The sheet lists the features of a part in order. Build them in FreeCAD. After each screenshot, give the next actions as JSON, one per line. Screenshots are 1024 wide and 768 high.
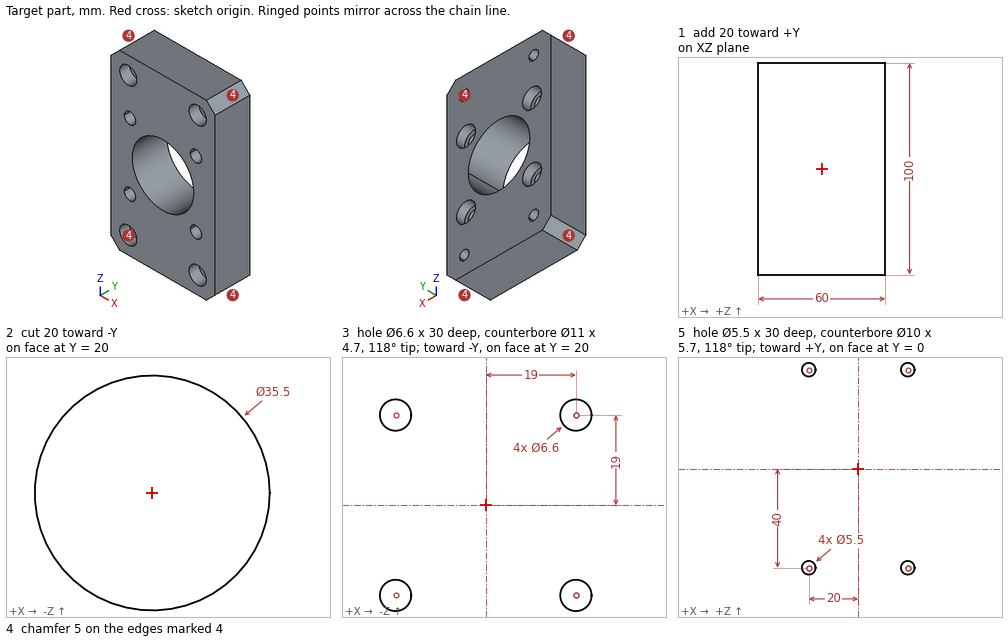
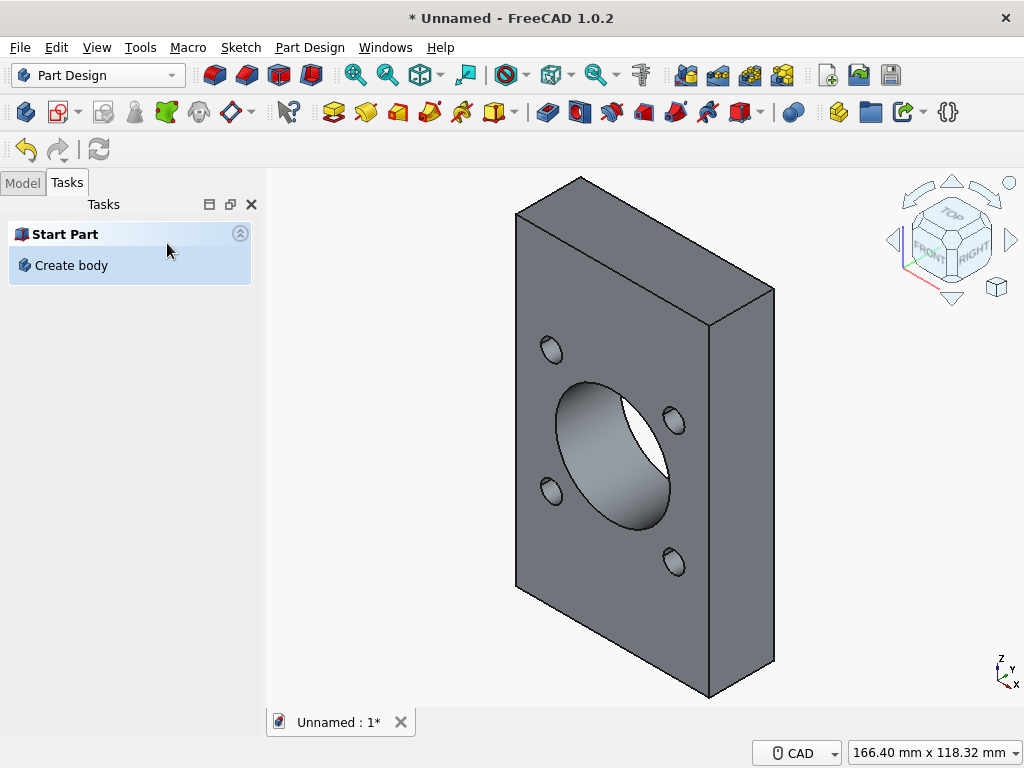
{"action": "left_click", "coordinate": [742, 306]}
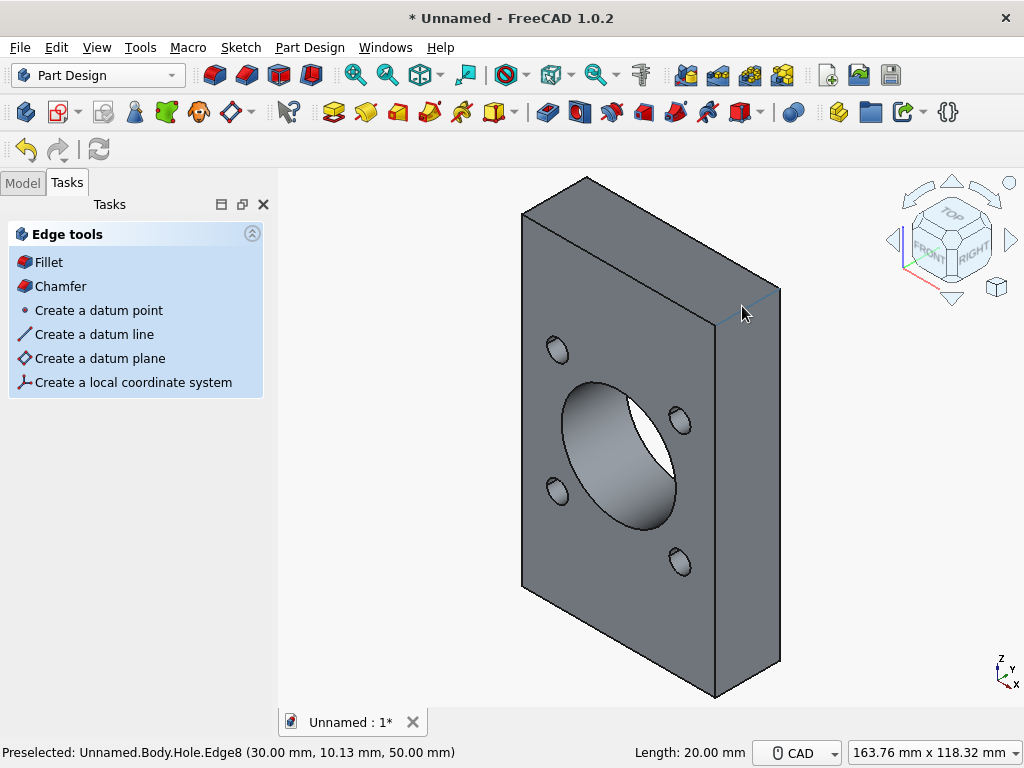
{"action": "key", "text": "2"}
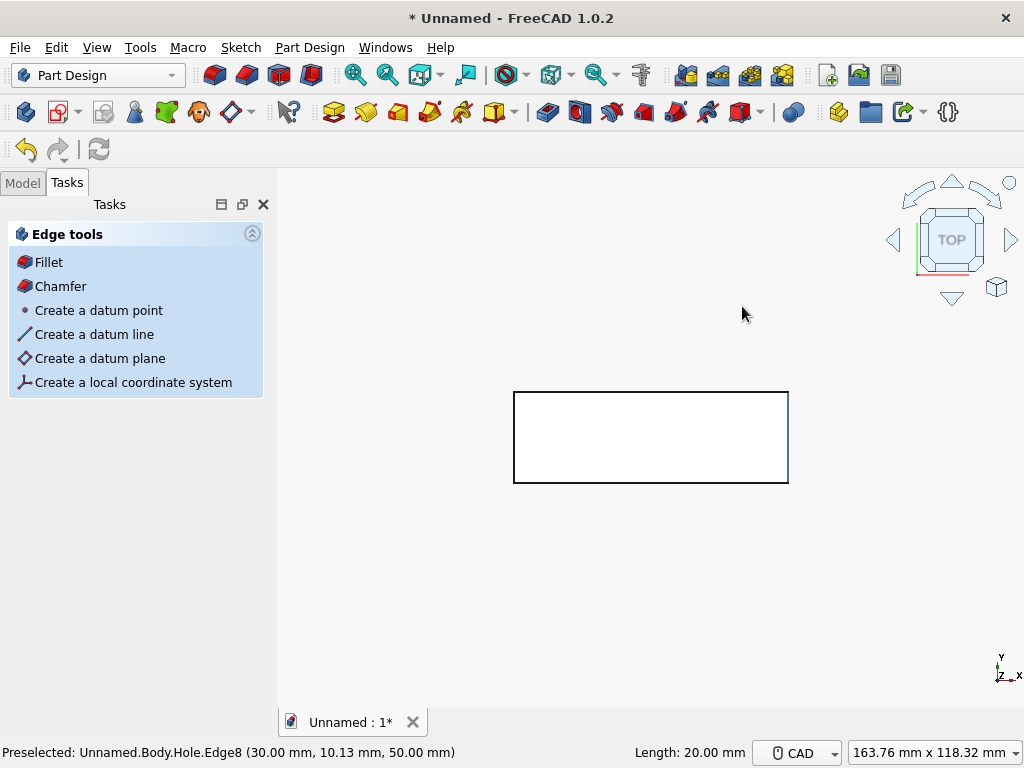
{"action": "left_click", "coordinate": [356, 76]}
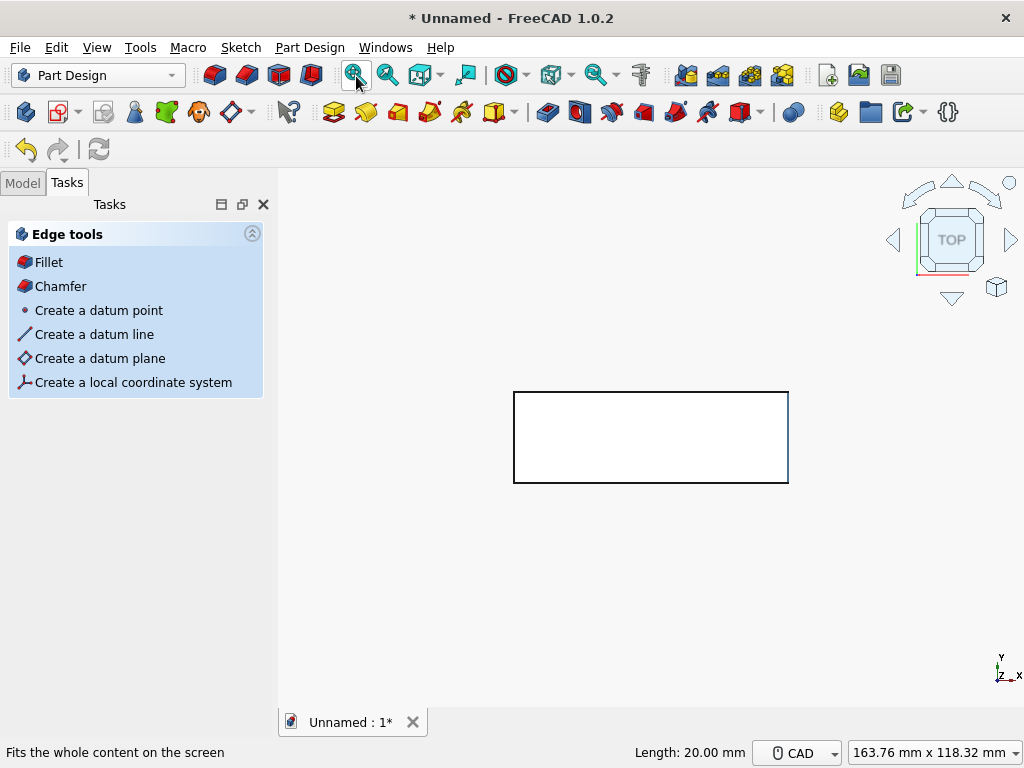
{"action": "left_click", "coordinate": [514, 436], "text": "ctrl"}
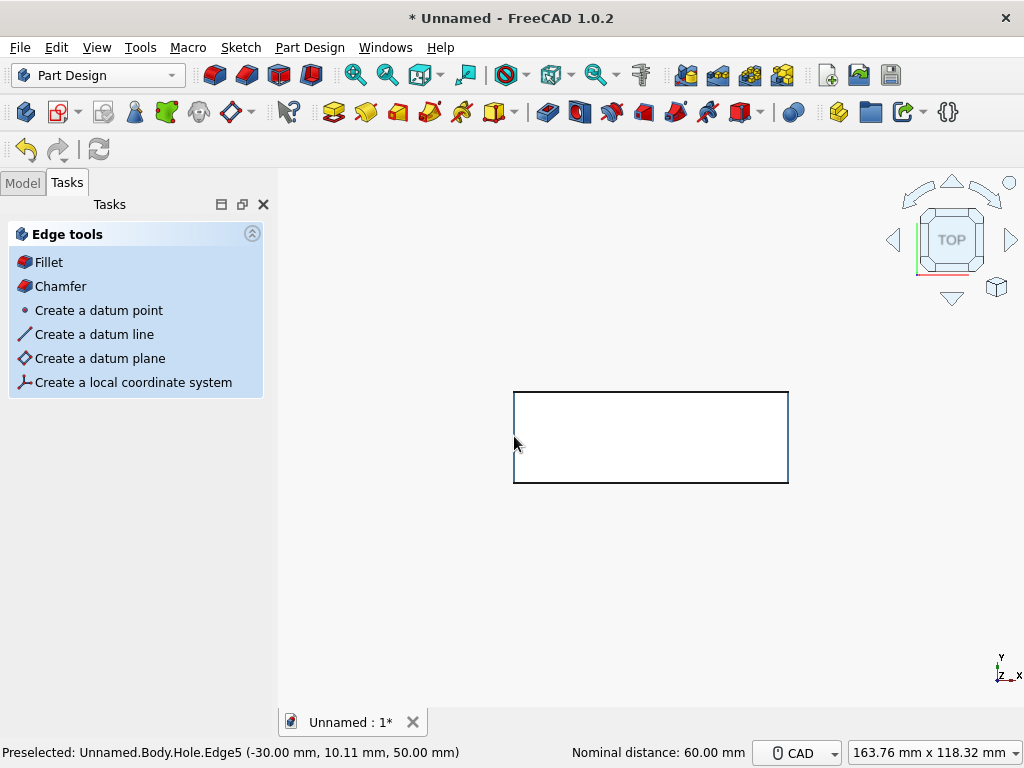
{"action": "key", "text": "1"}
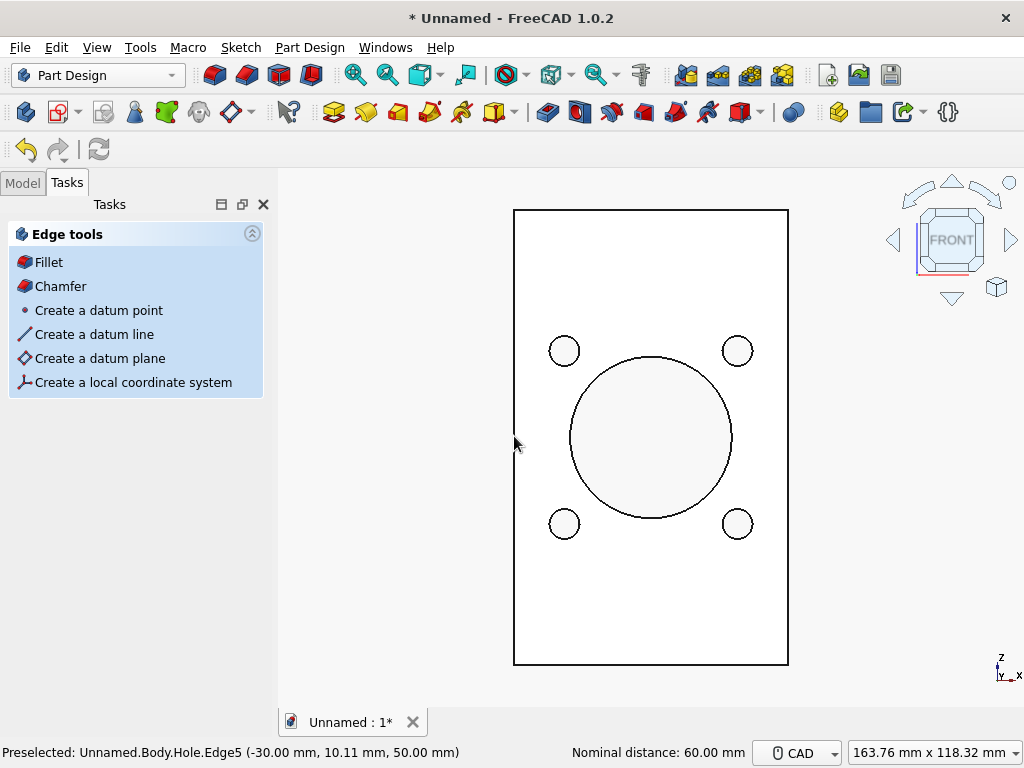
{"action": "key", "text": "3"}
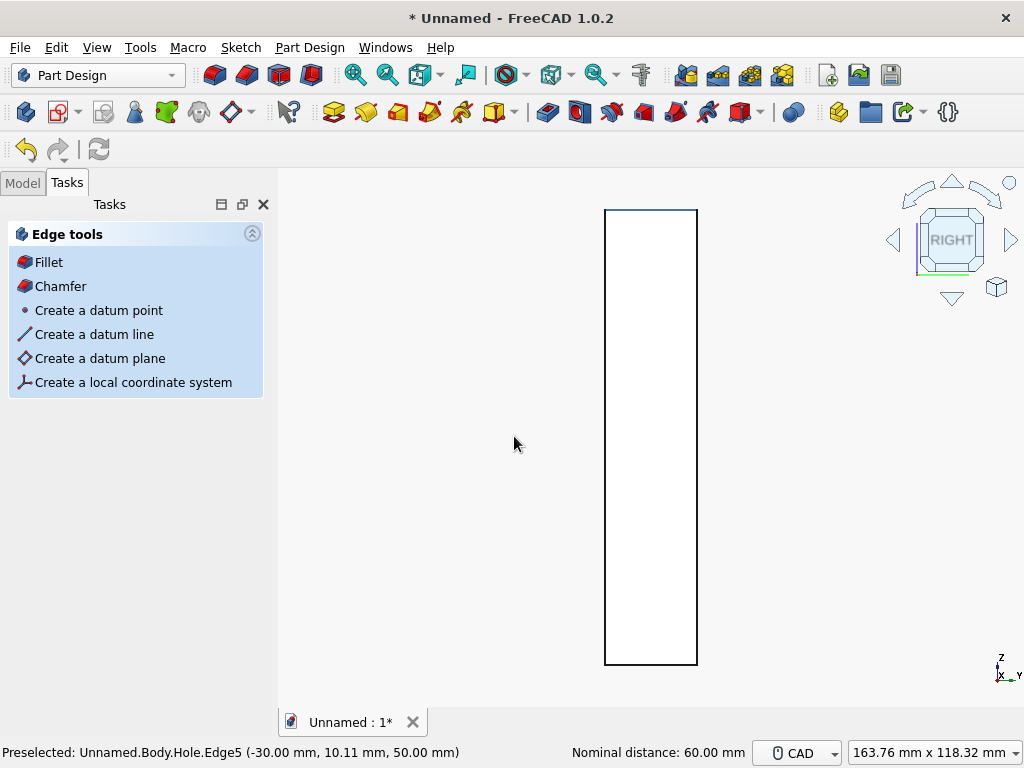
{"action": "left_click", "coordinate": [651, 664], "text": "ctrl"}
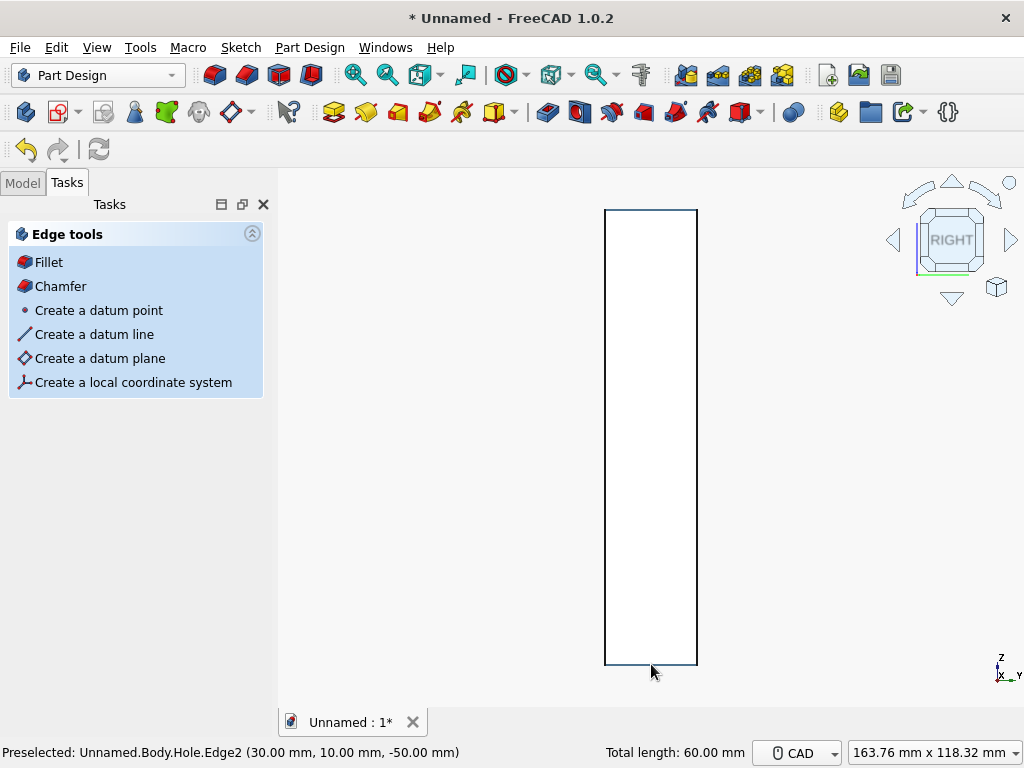
{"action": "key", "text": "5"}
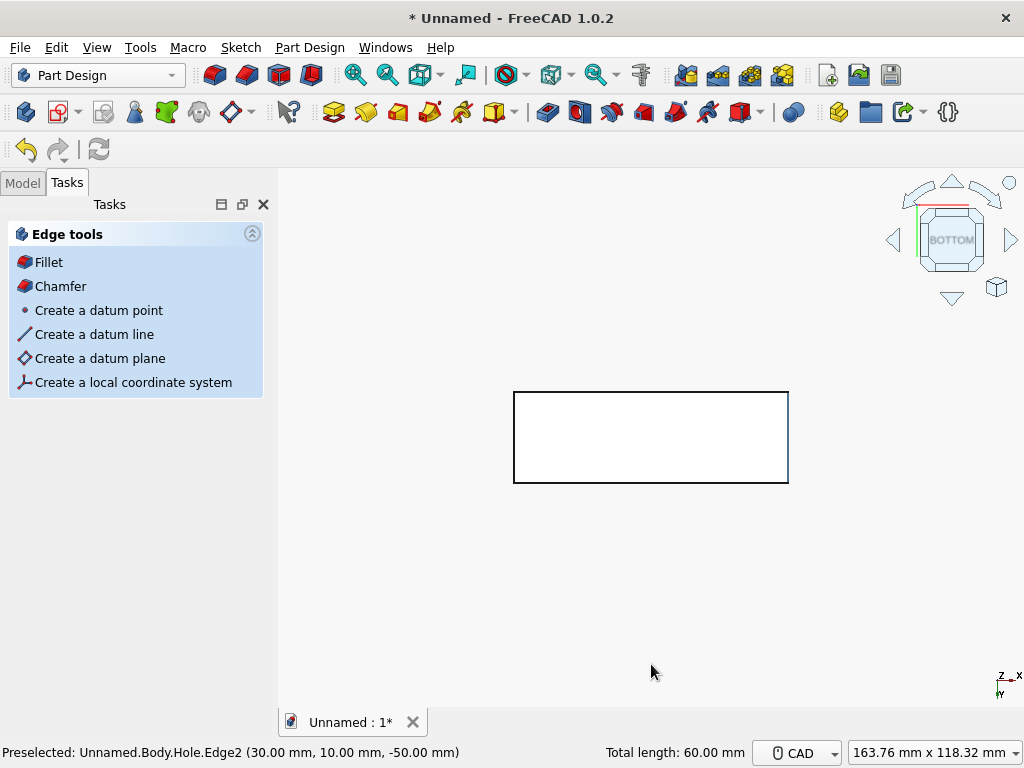
{"action": "left_click", "coordinate": [356, 76]}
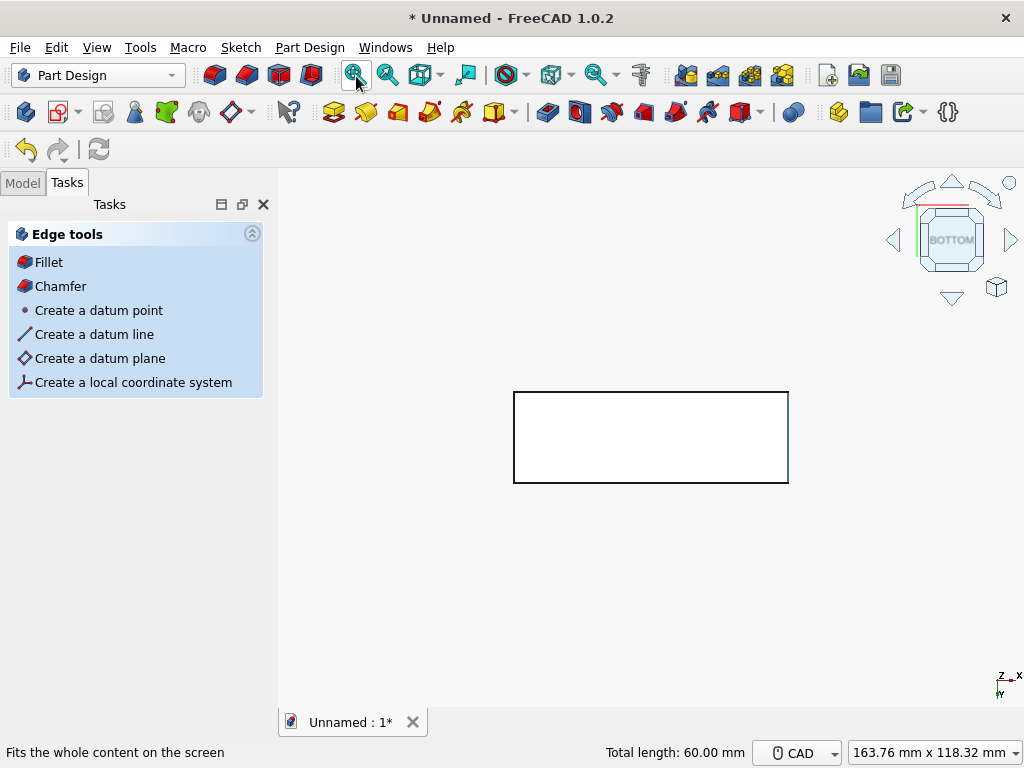
{"action": "left_click", "coordinate": [514, 436], "text": "ctrl"}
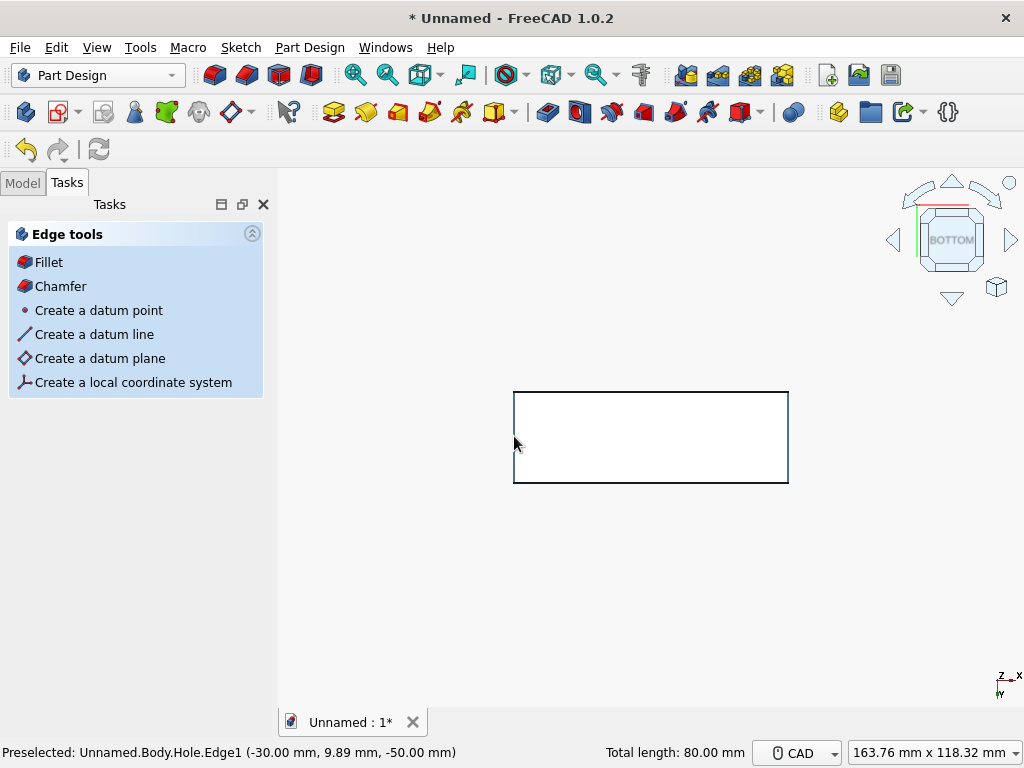
{"action": "left_click", "coordinate": [248, 76]}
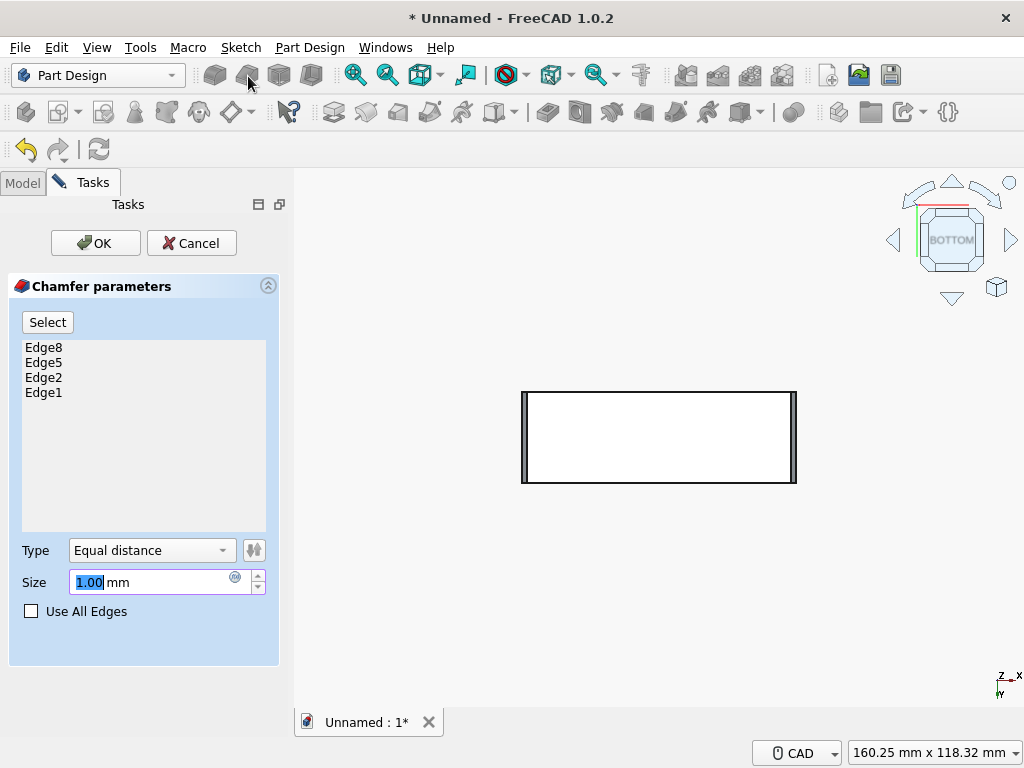
{"action": "type", "text": "5"}
{"action": "key", "text": "Tab"}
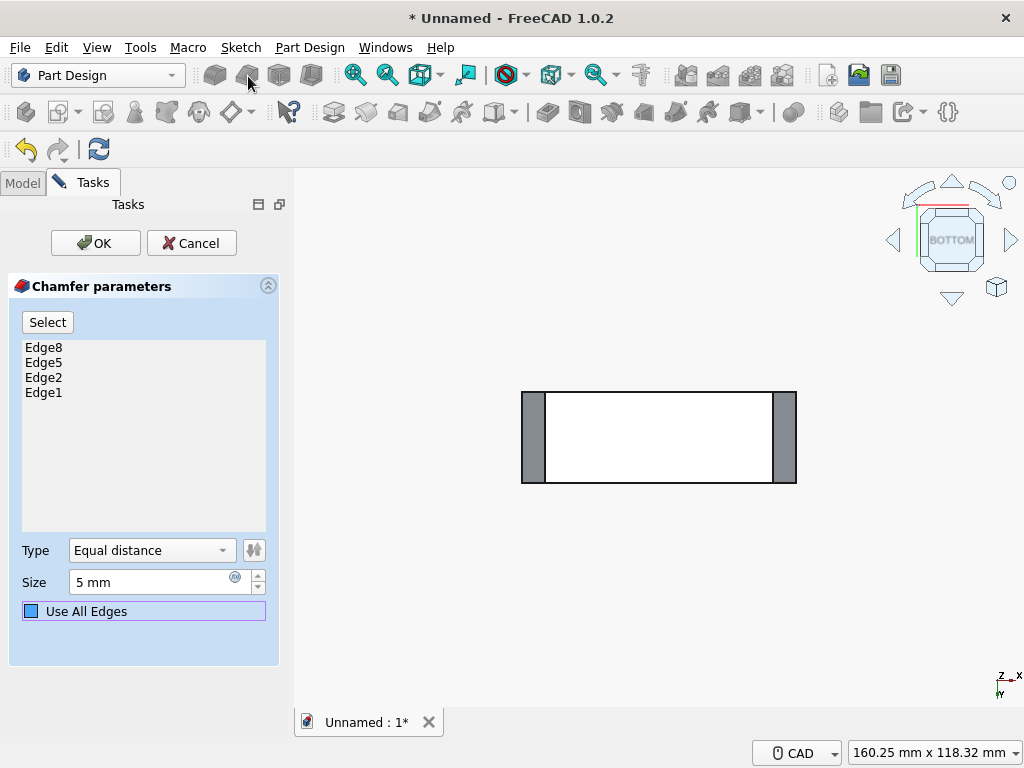
{"action": "left_click", "coordinate": [96, 243]}